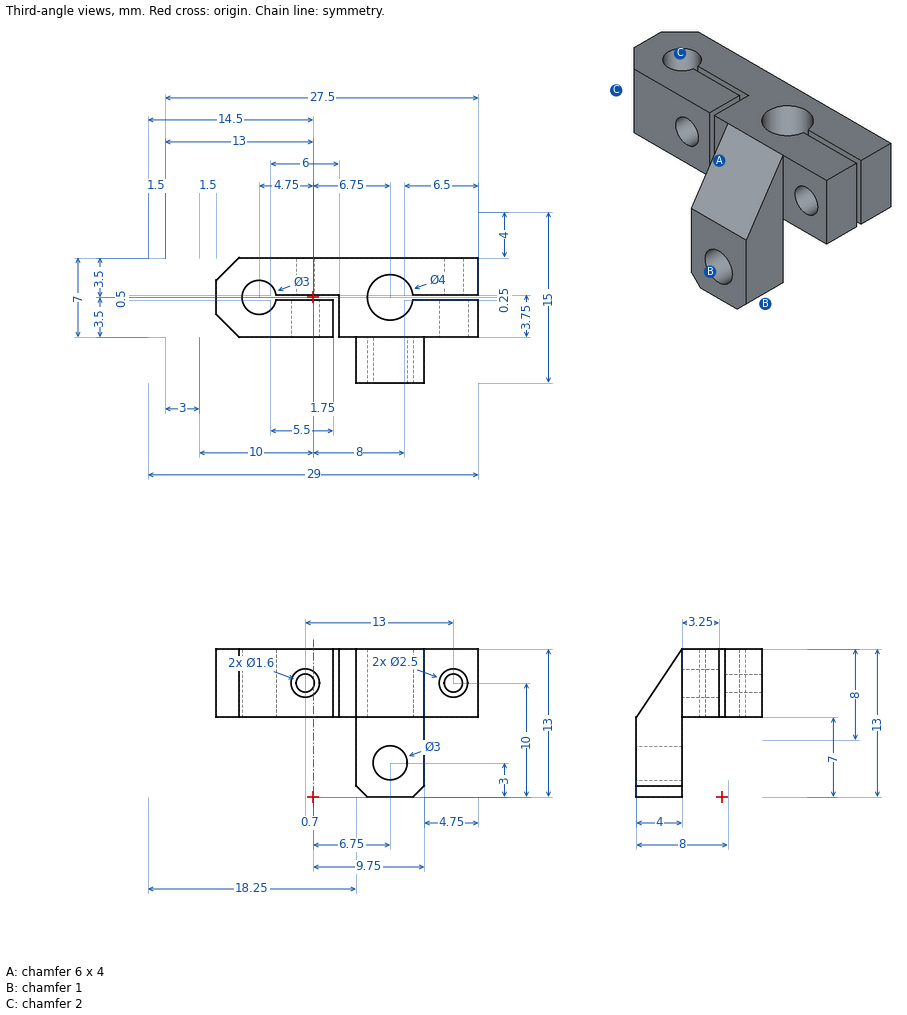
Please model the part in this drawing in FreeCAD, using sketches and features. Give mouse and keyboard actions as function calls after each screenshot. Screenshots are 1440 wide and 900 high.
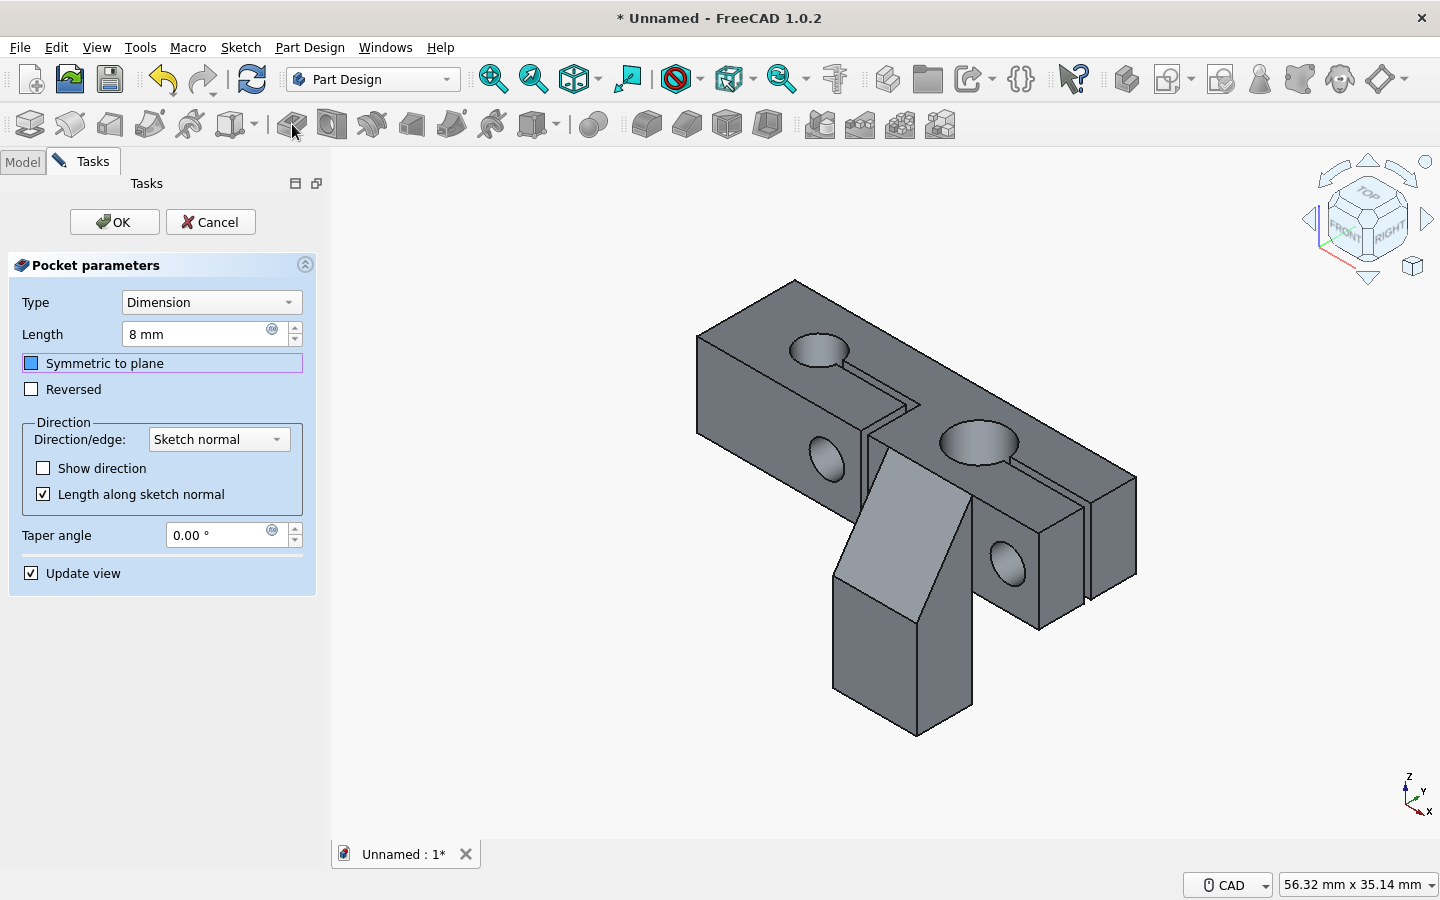
click(115, 222)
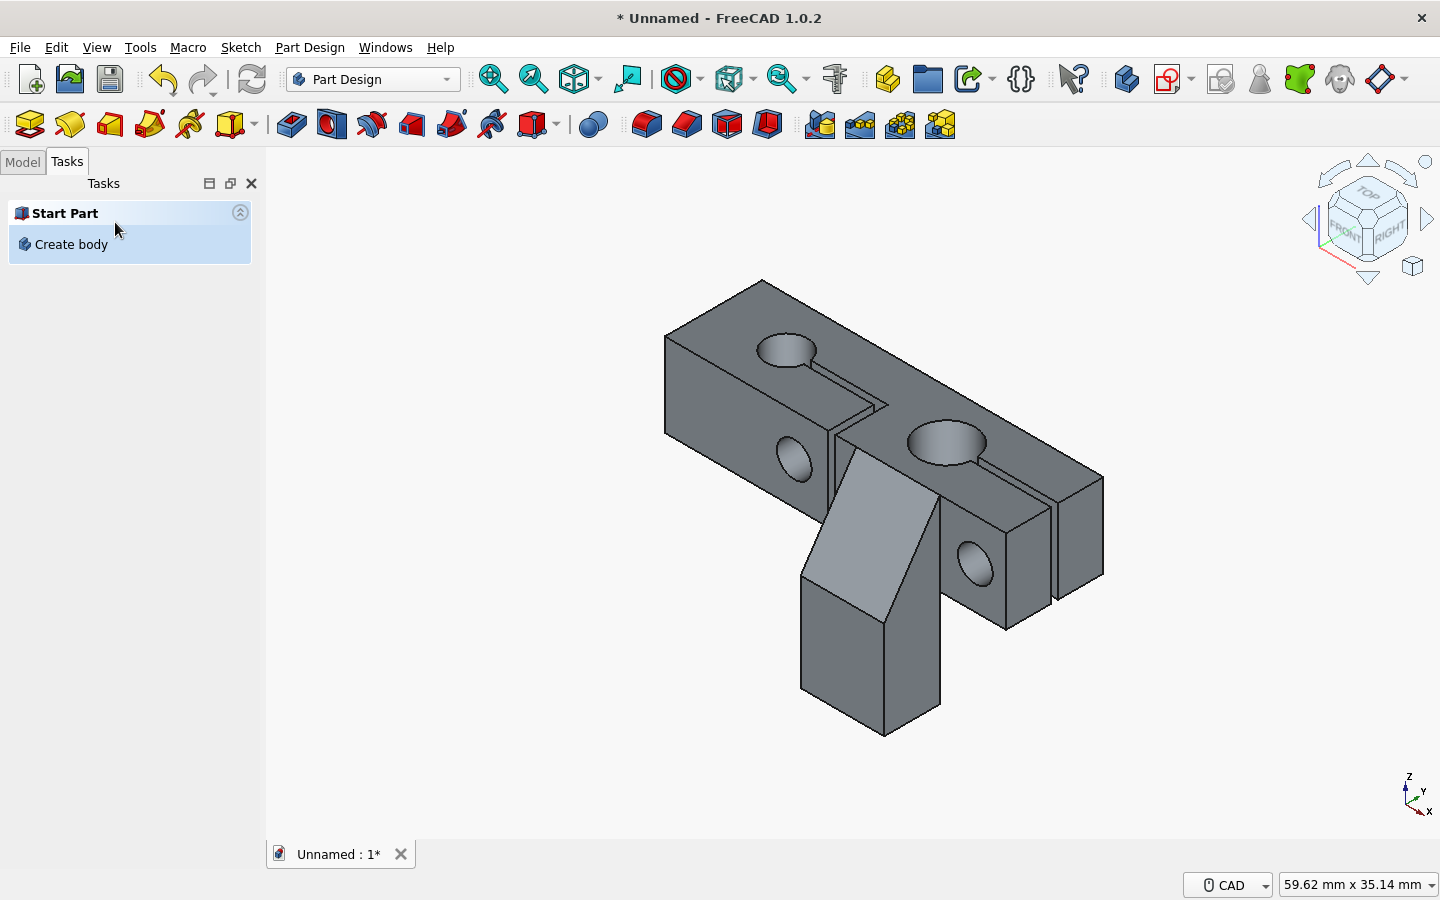
click(842, 655)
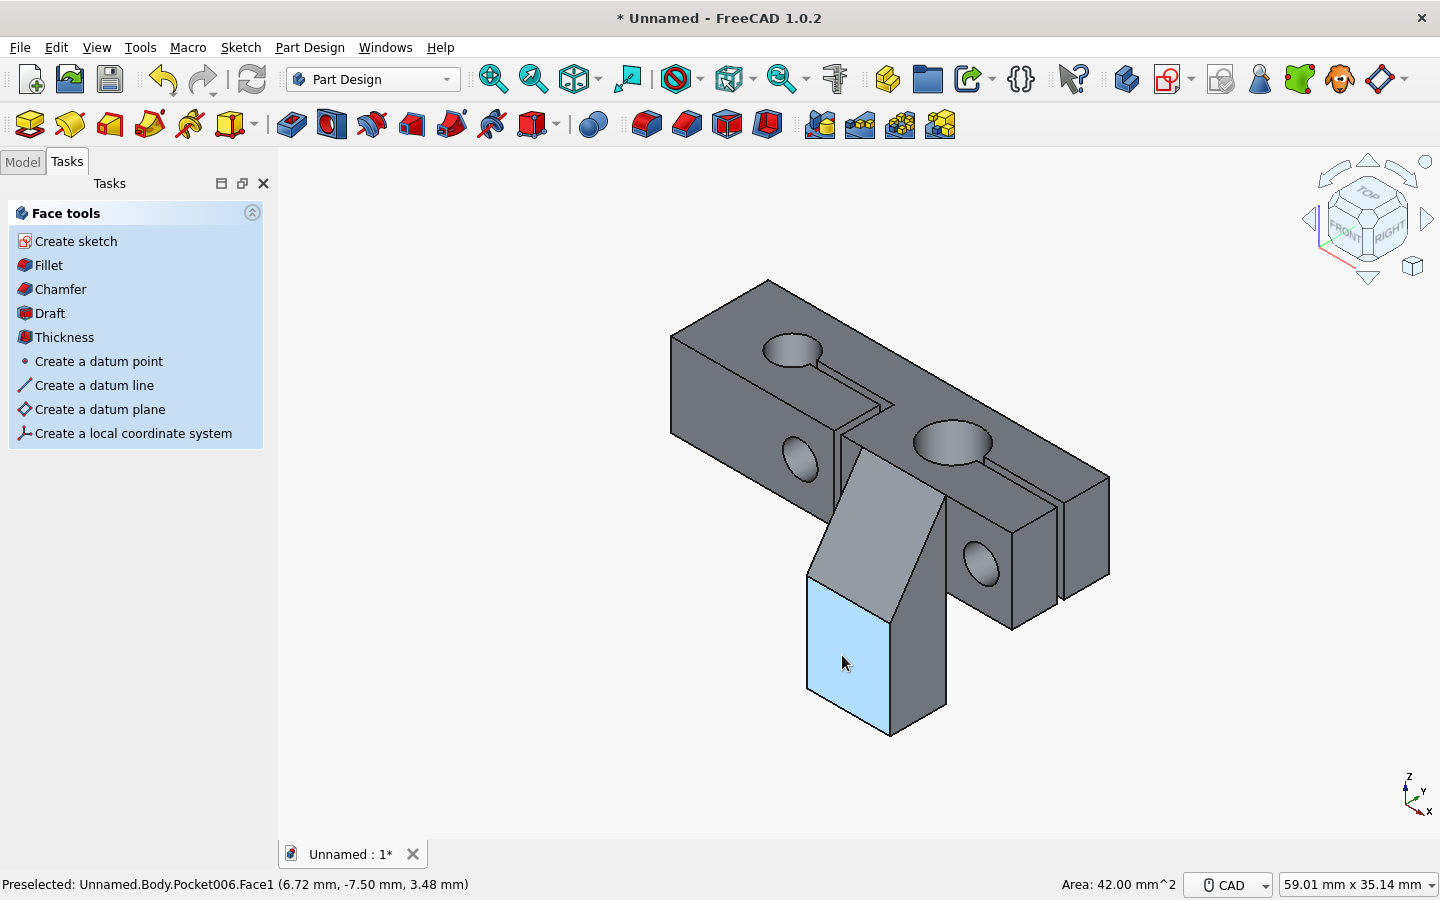
click(1168, 80)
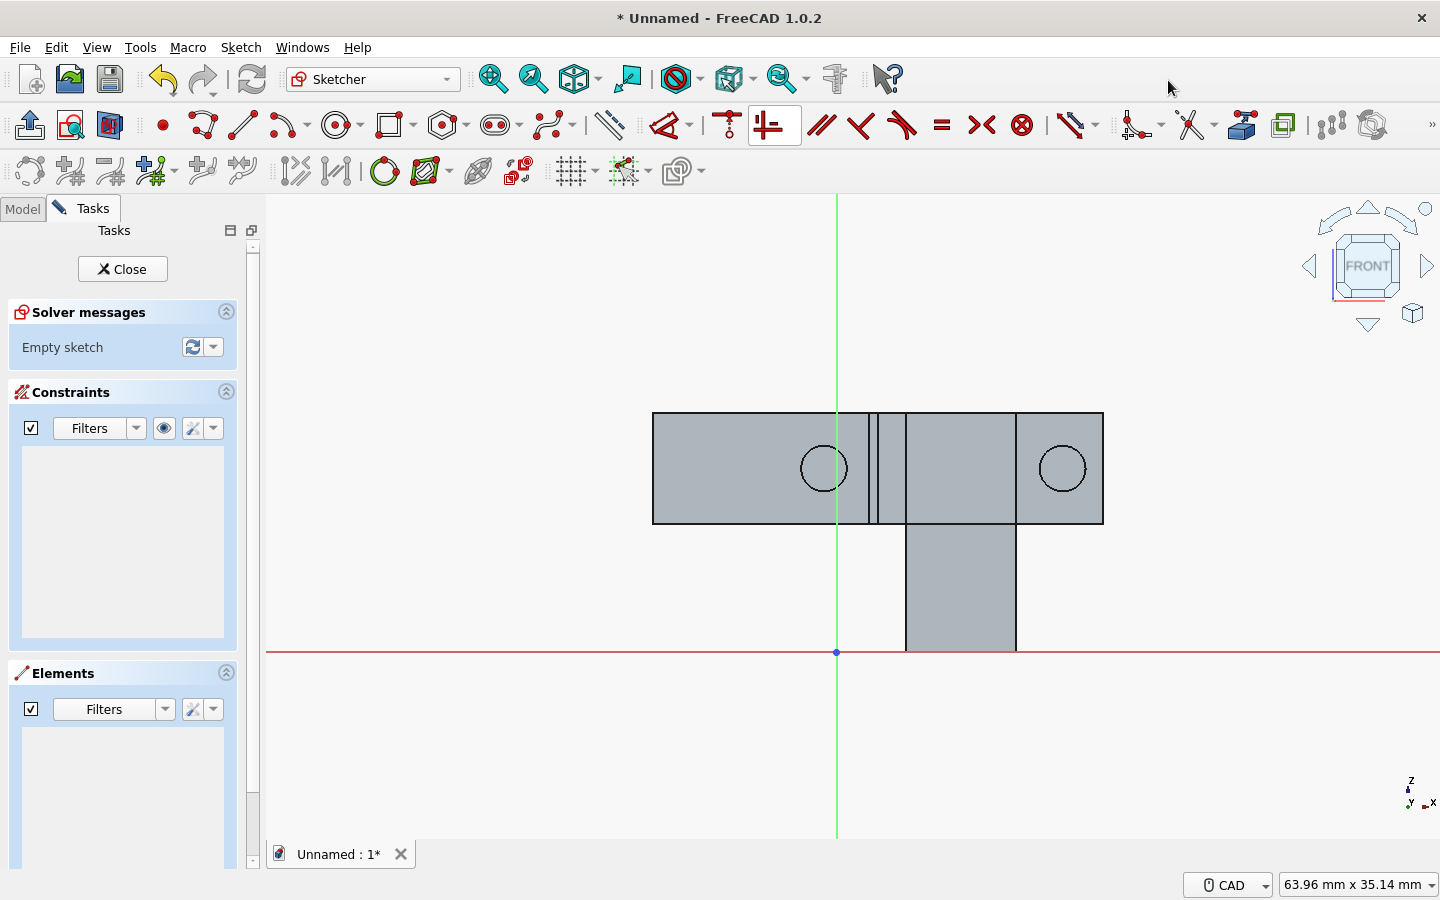
scroll(988, 610, up, 10)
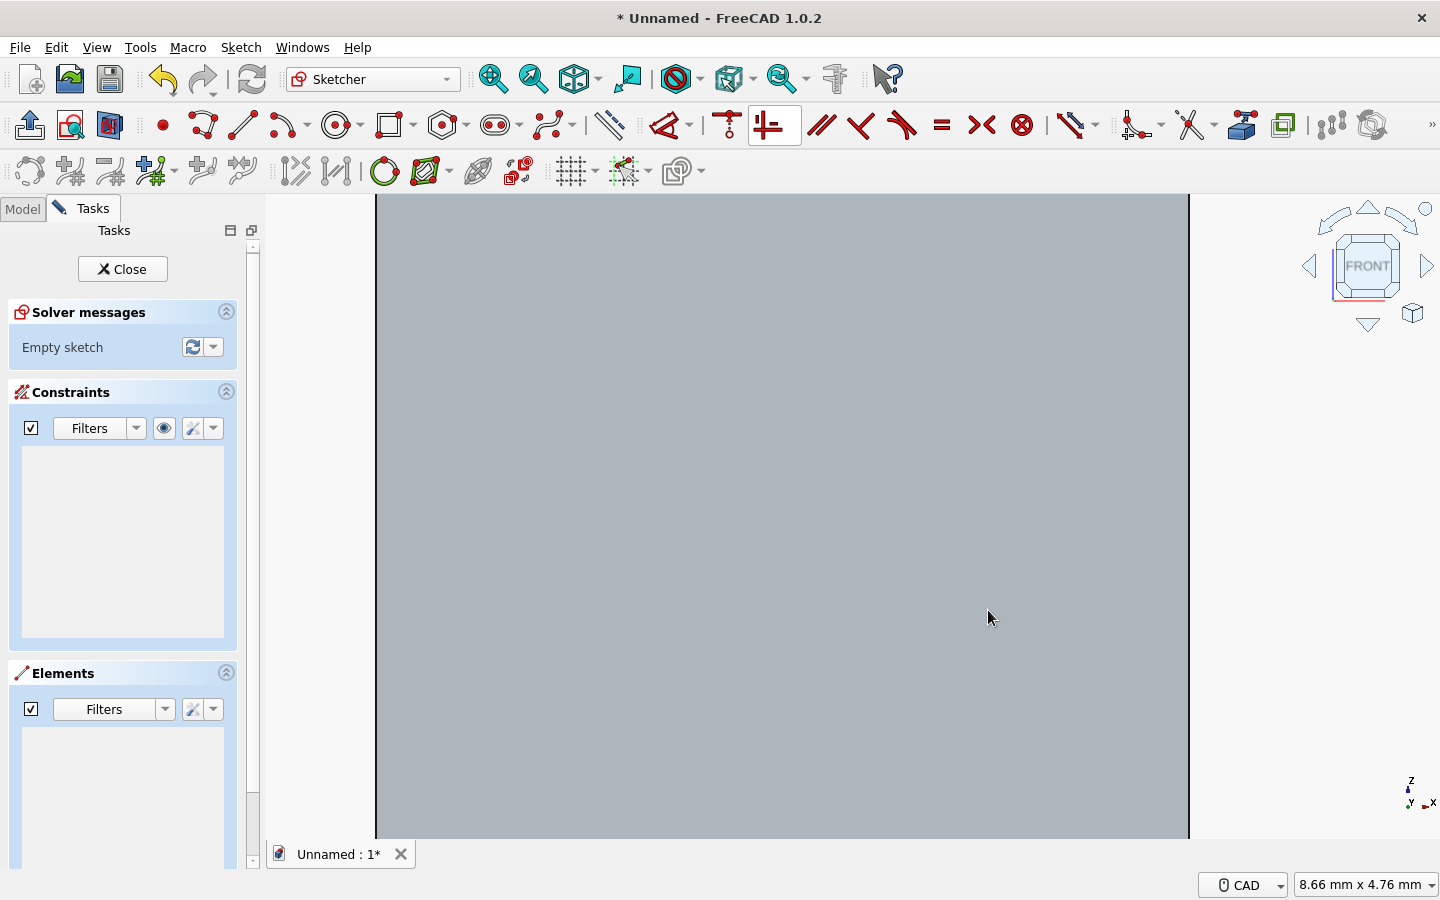
click(336, 126)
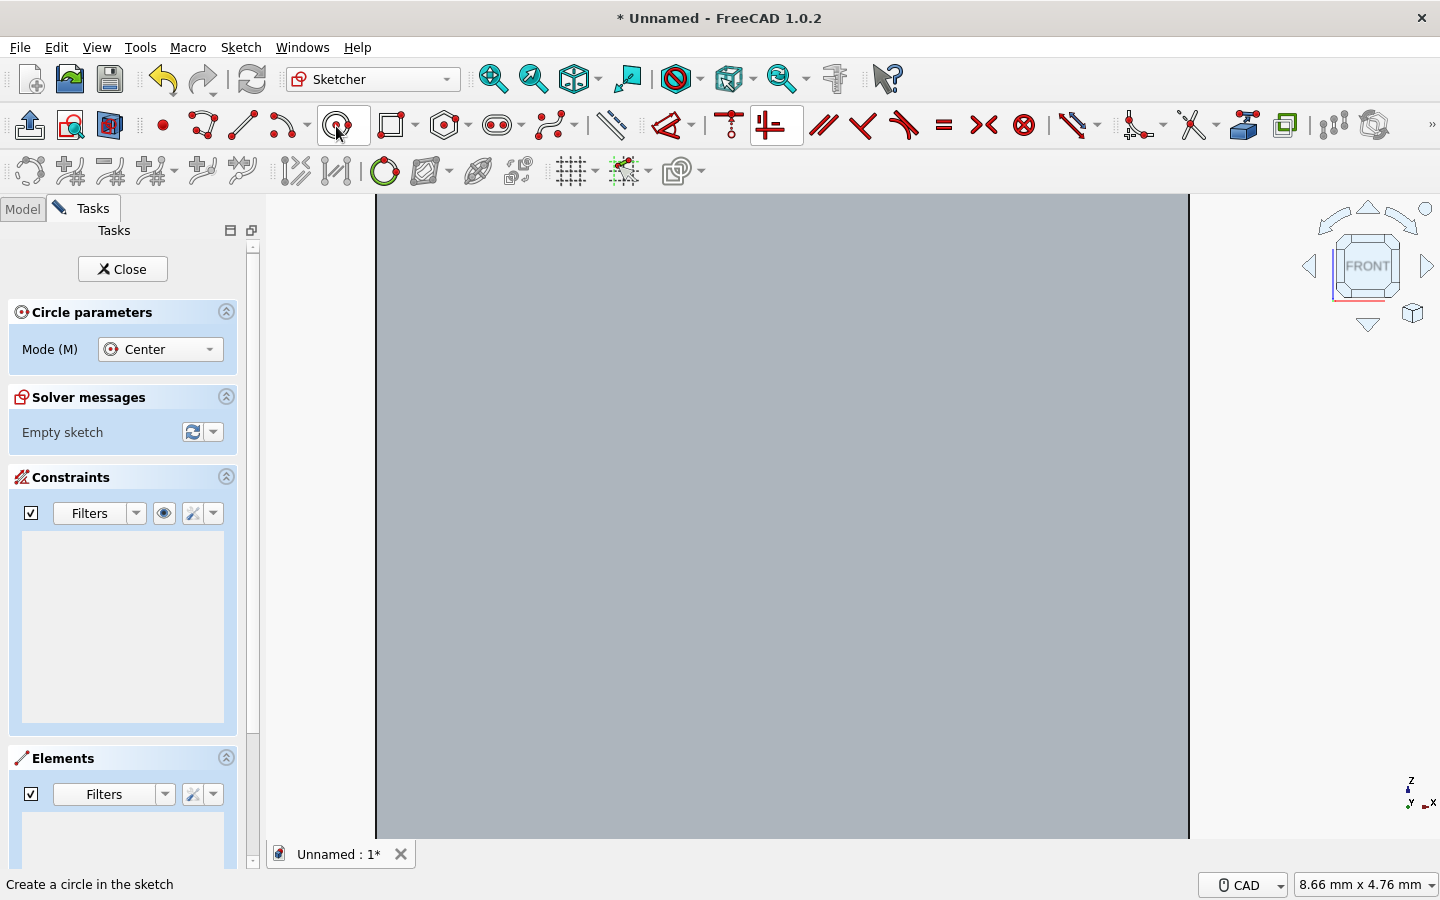
click(782, 510)
move(926, 366)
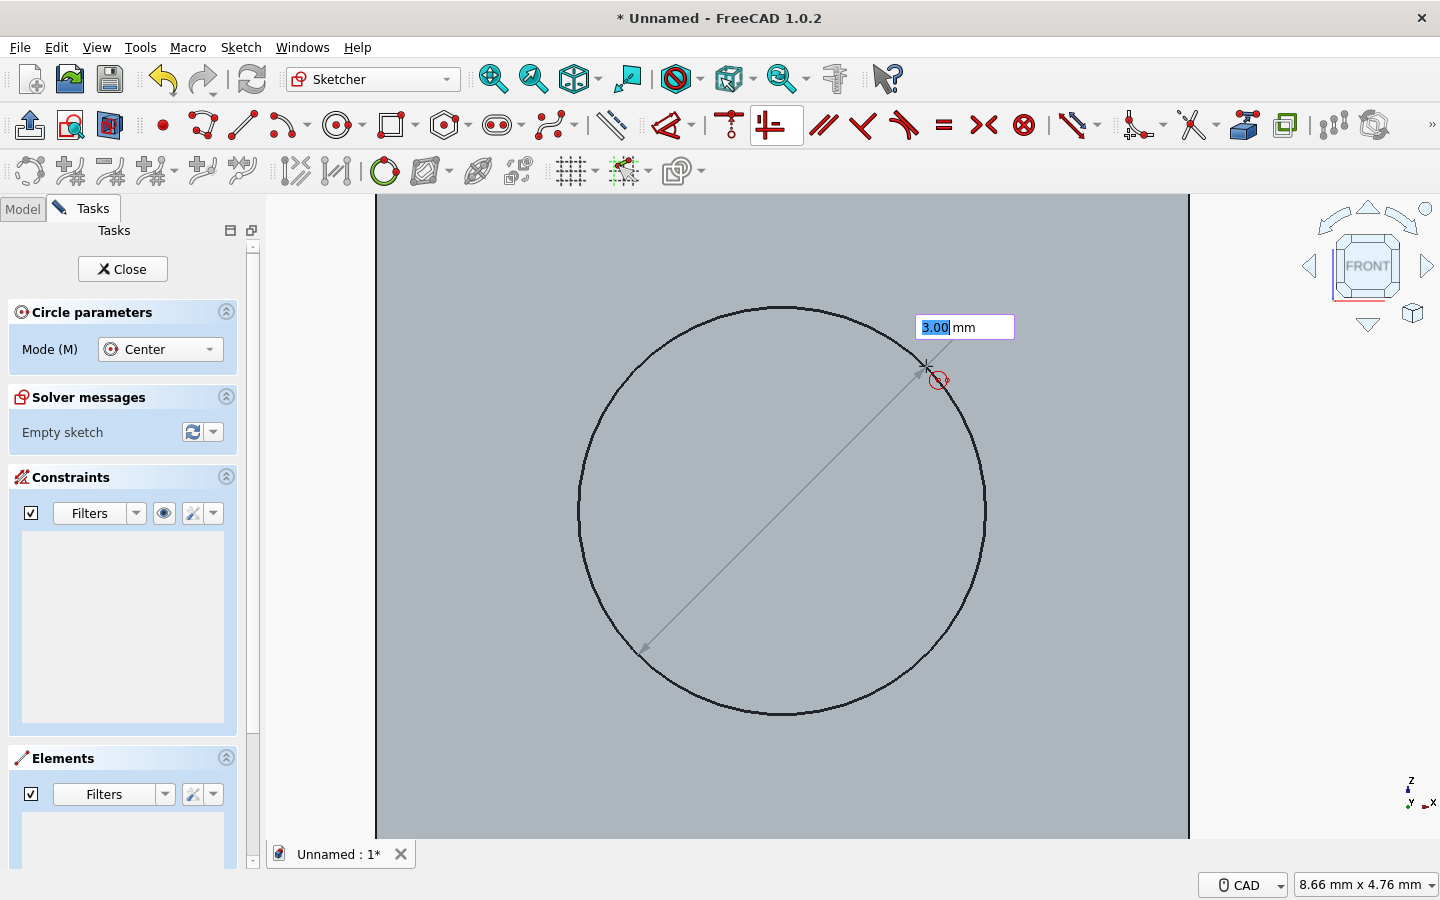
text(3)
key(Return)
key(Escape)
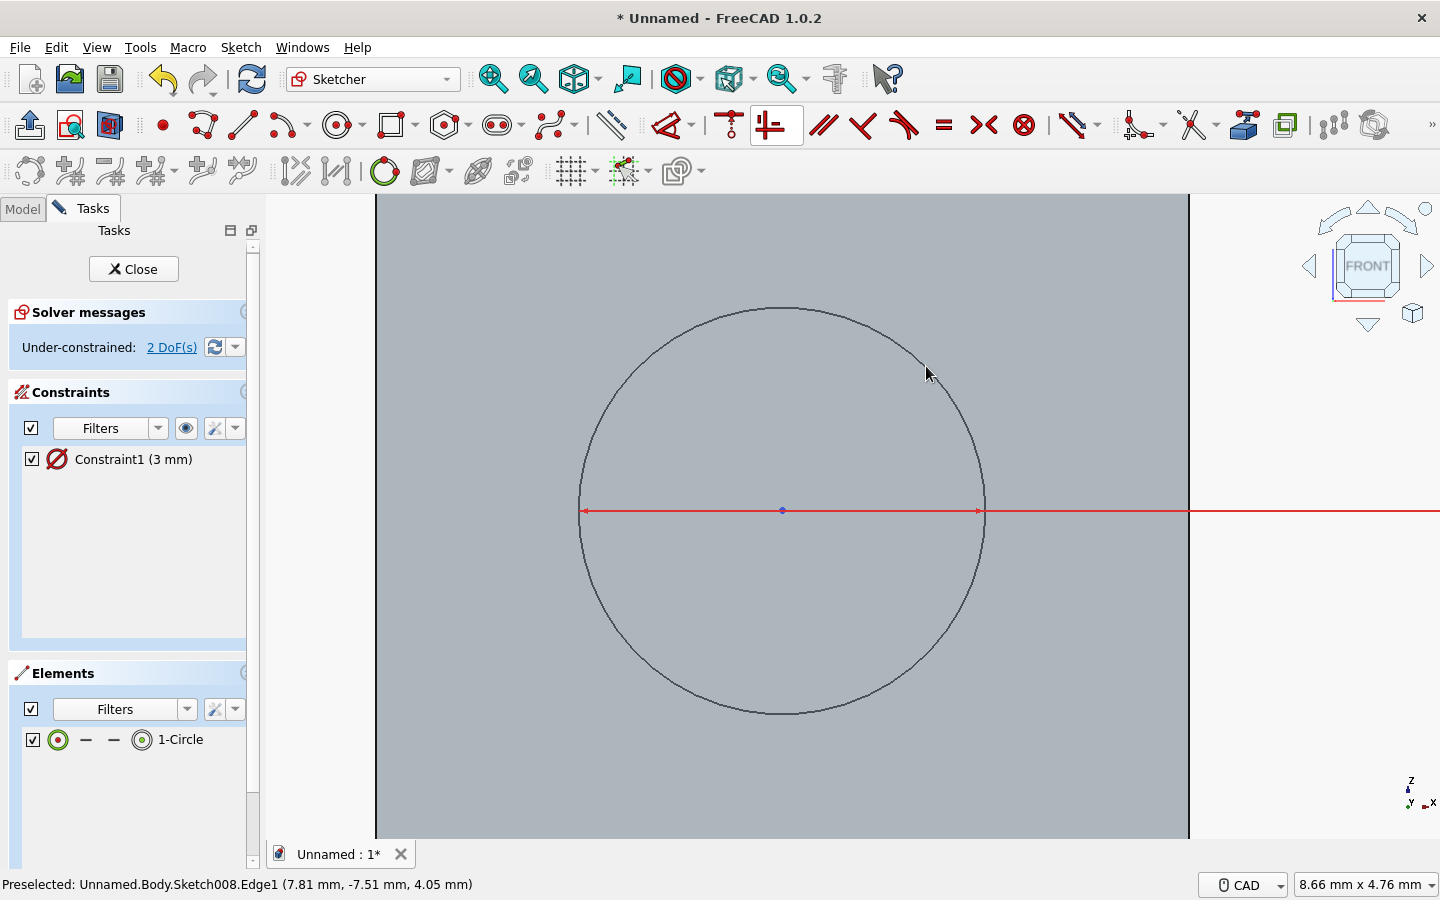
click(666, 126)